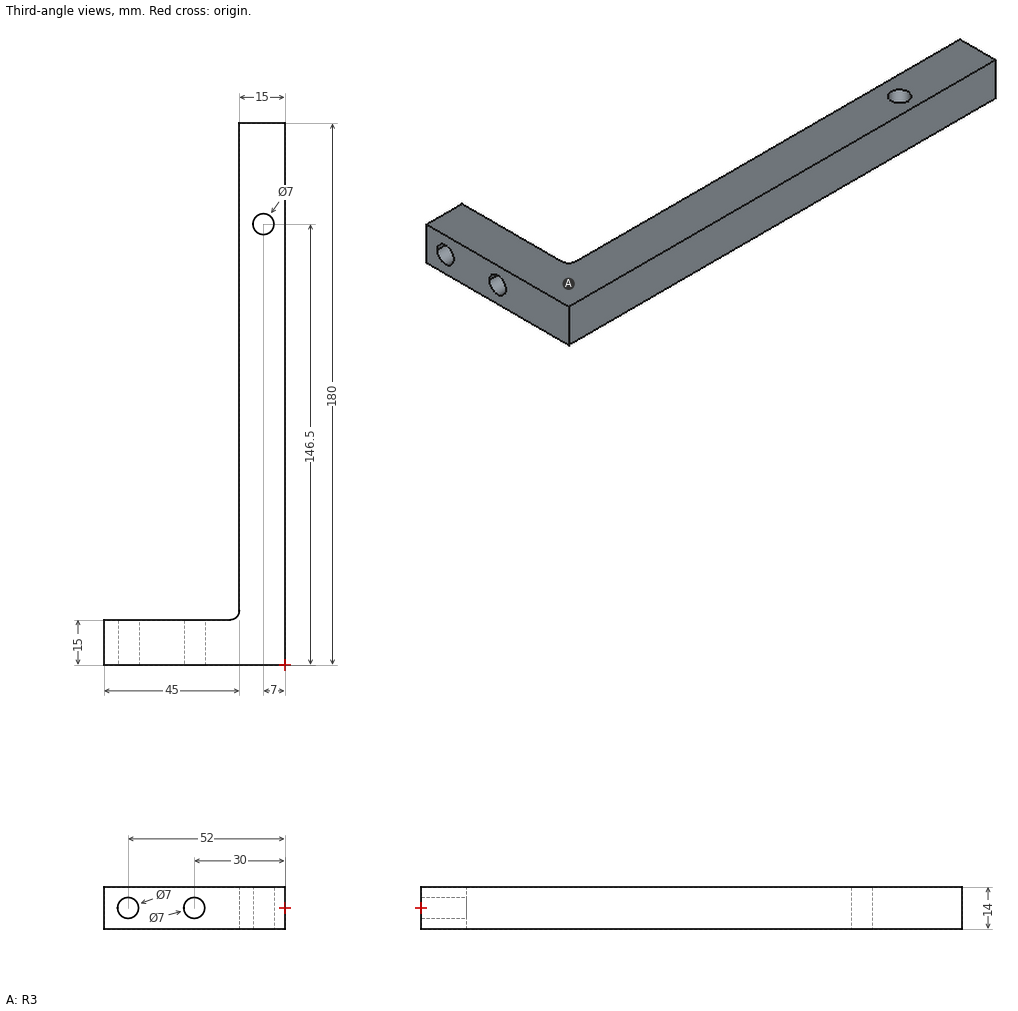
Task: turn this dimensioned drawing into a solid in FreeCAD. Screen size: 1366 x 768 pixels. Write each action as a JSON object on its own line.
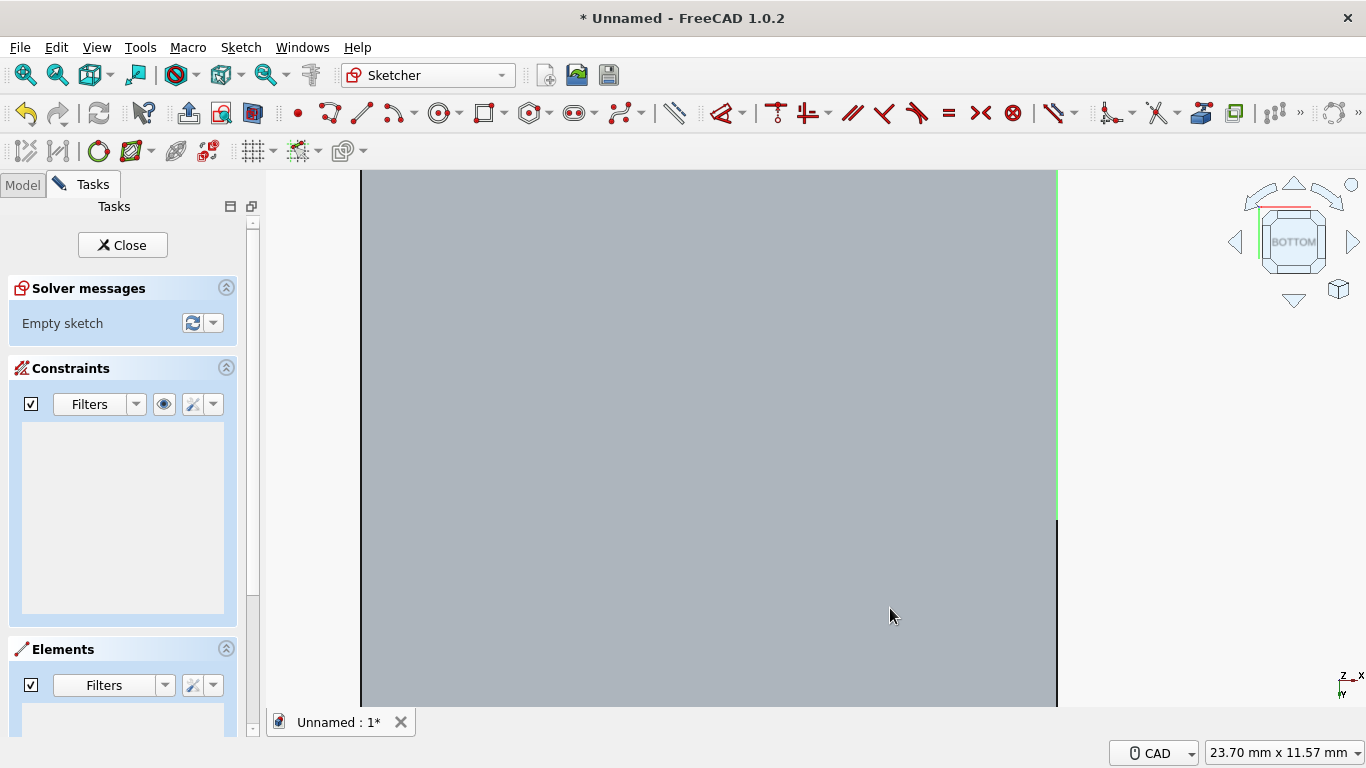
{"action": "left_click", "coordinate": [440, 114]}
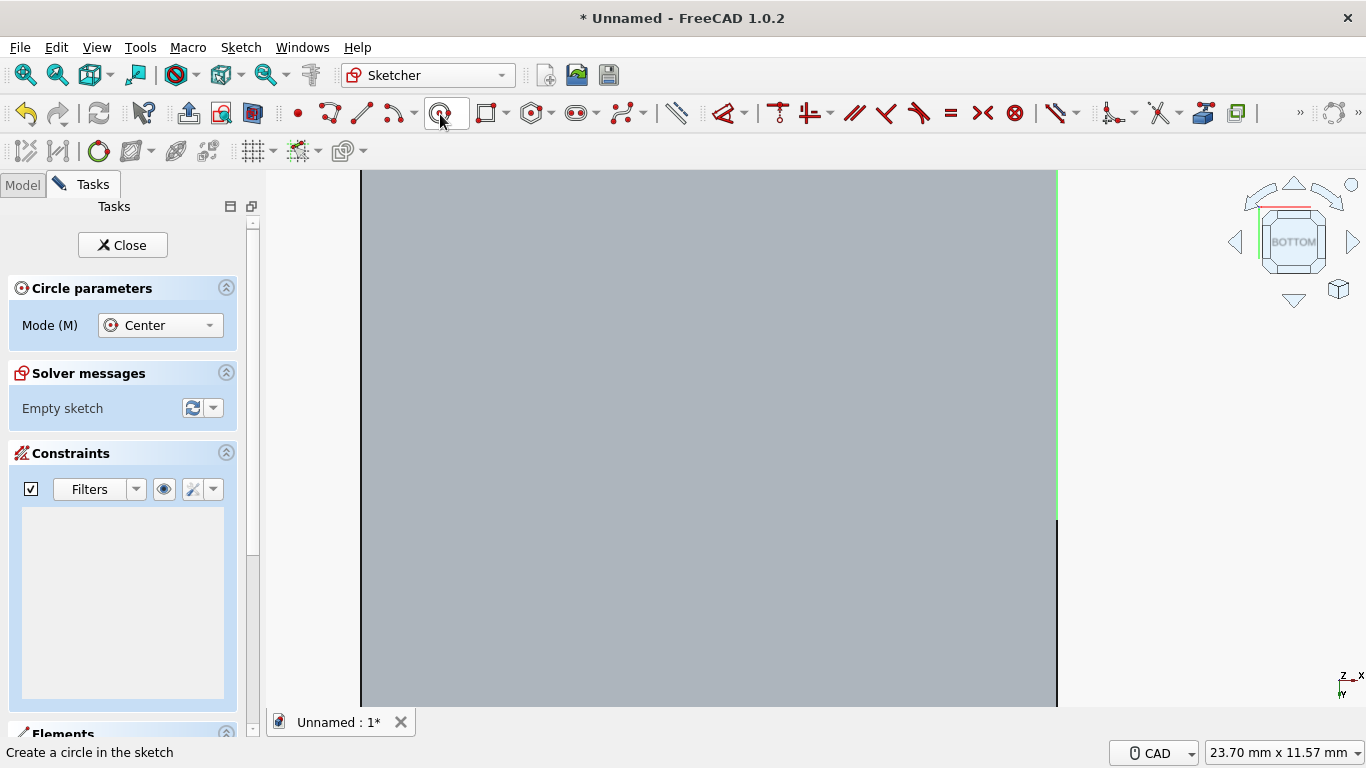
{"action": "left_click", "coordinate": [732, 431]}
{"action": "mouse_move", "coordinate": [847, 316]}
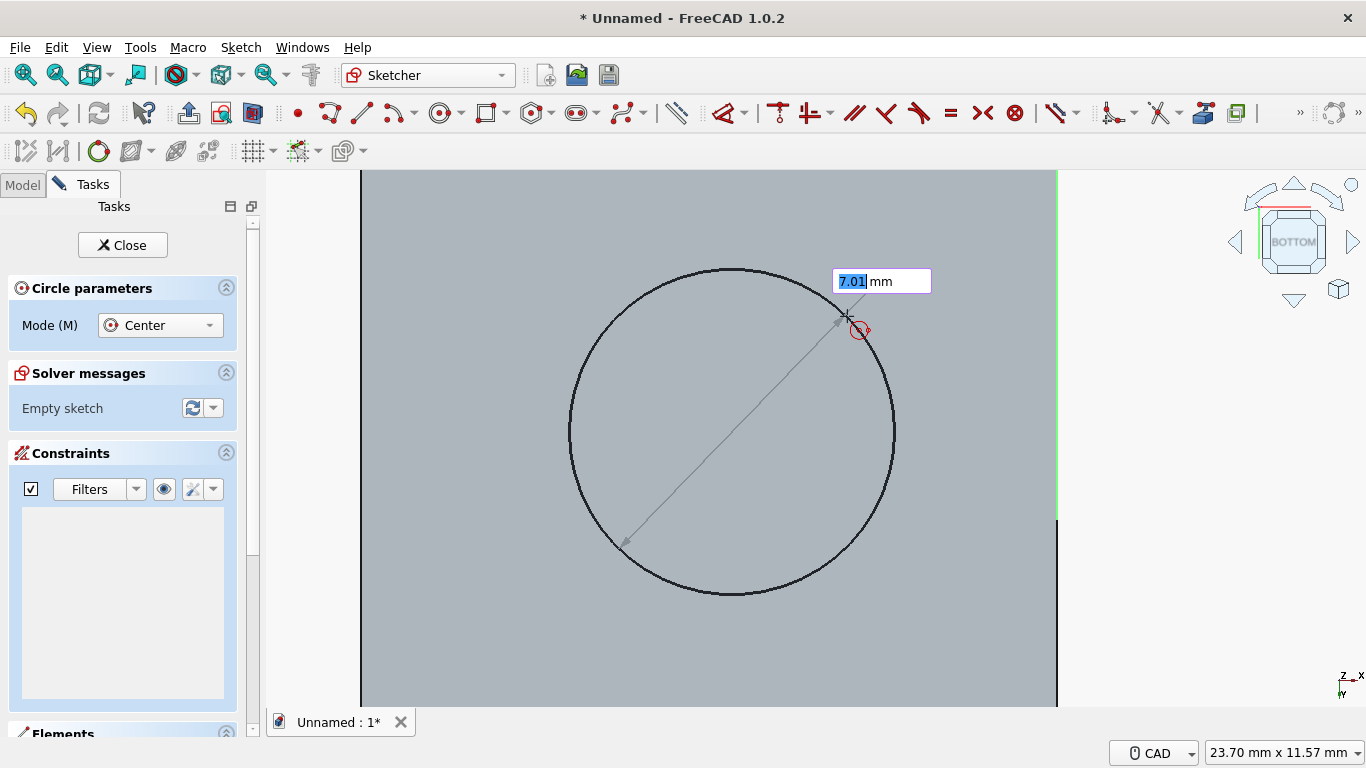
{"action": "type", "text": "7"}
{"action": "key", "text": "Return"}
{"action": "key", "text": "Escape"}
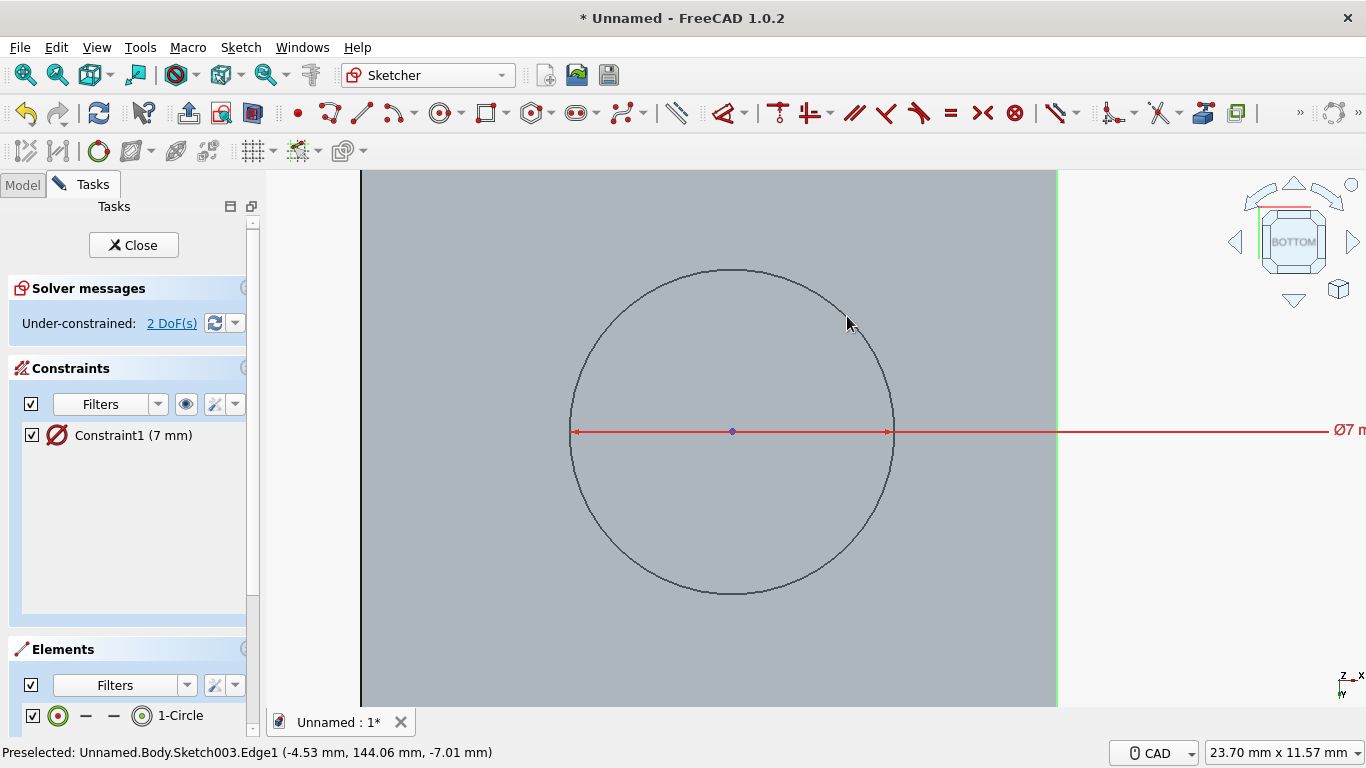
{"action": "left_click", "coordinate": [724, 114]}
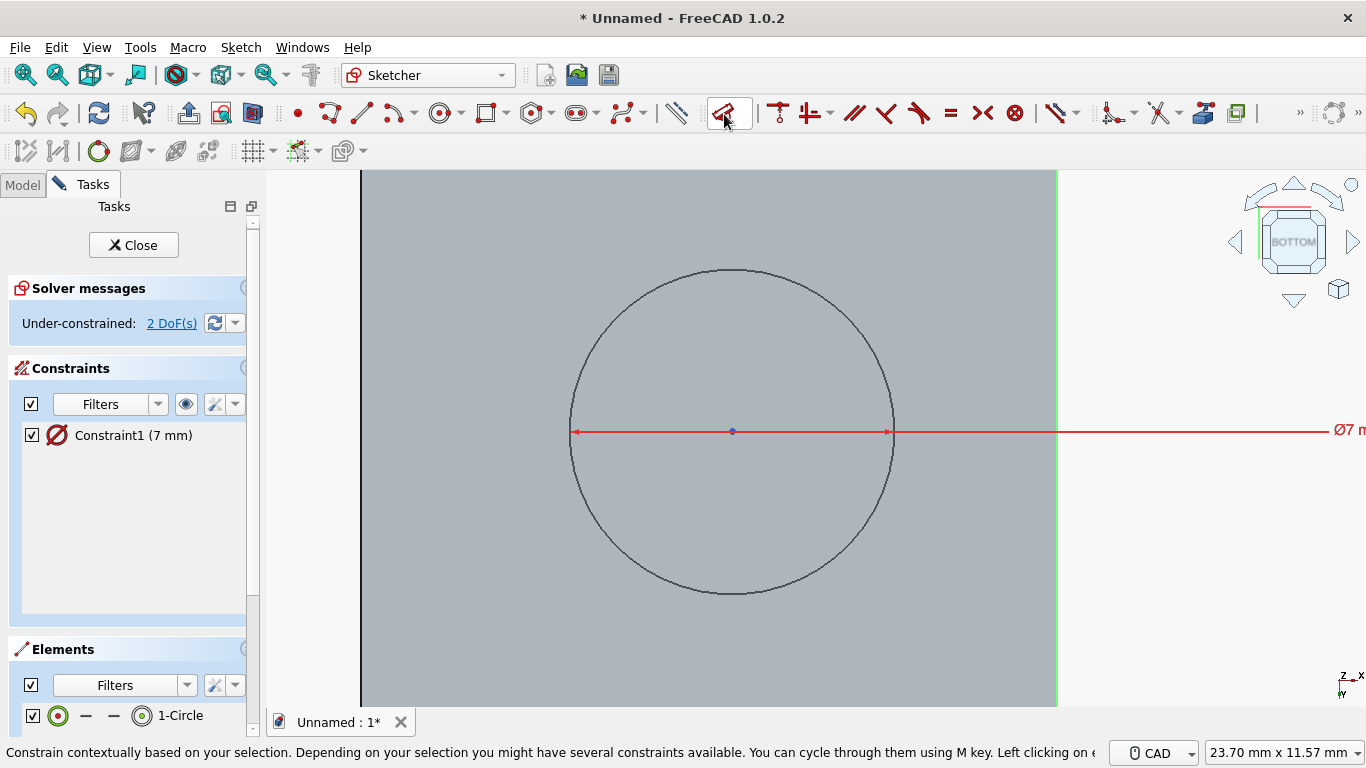
{"action": "left_click", "coordinate": [732, 432]}
{"action": "left_click", "coordinate": [820, 466]}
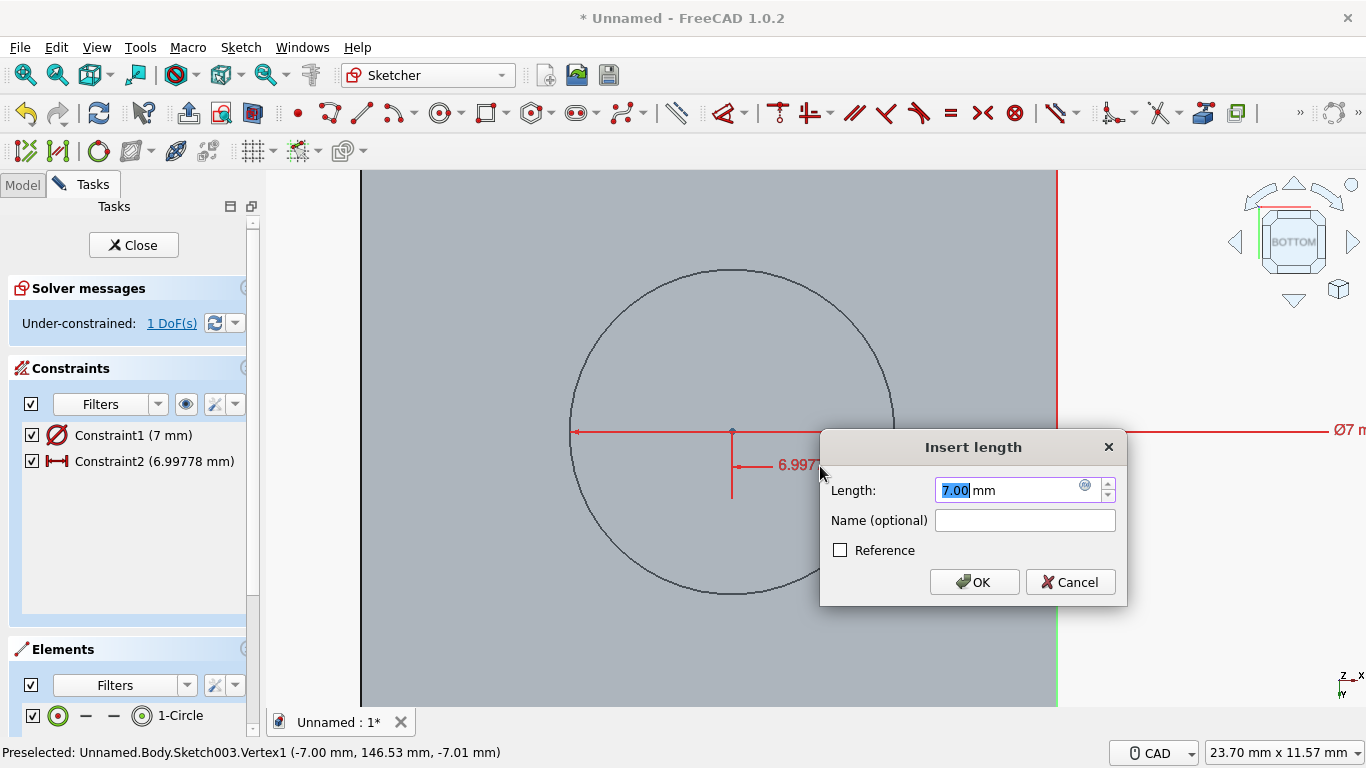
{"action": "type", "text": "7"}
{"action": "key", "text": "Return"}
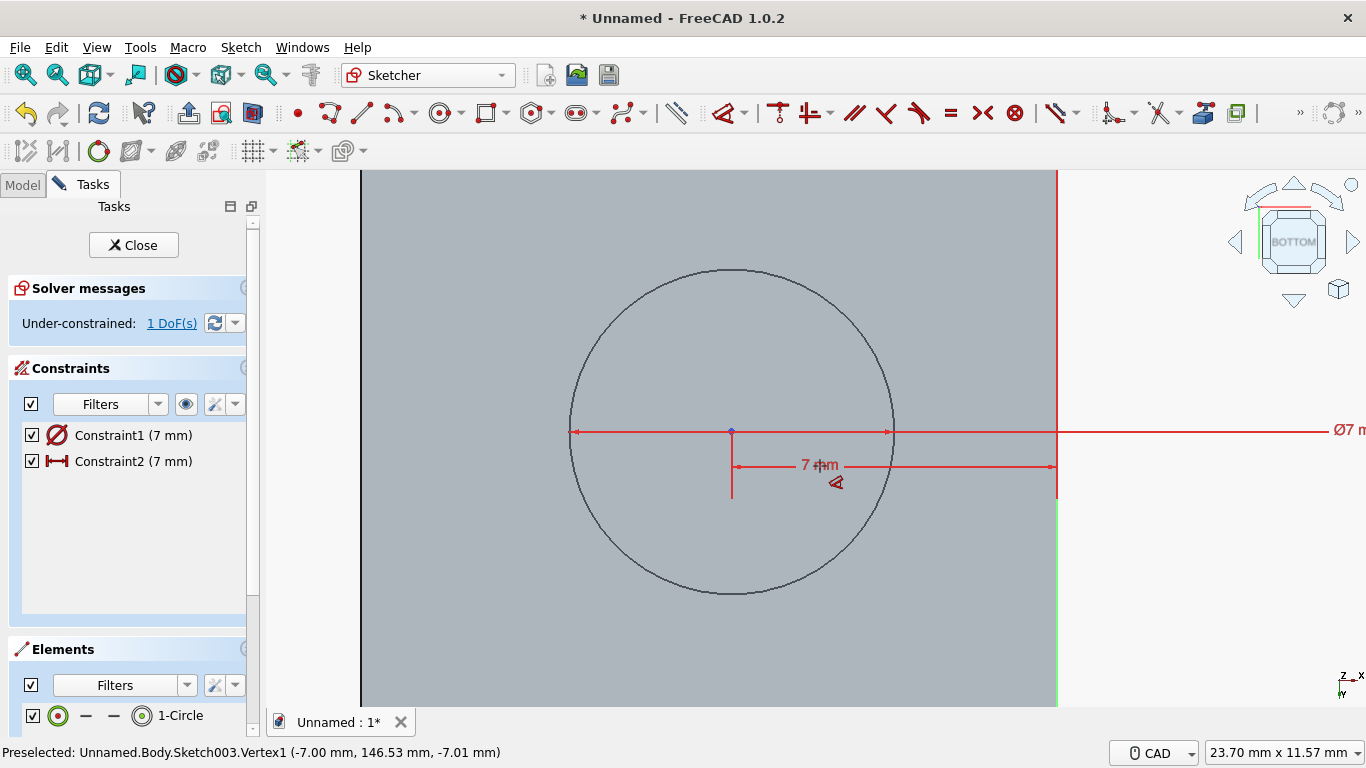
{"action": "left_click", "coordinate": [732, 432]}
{"action": "left_click", "coordinate": [1091, 315]}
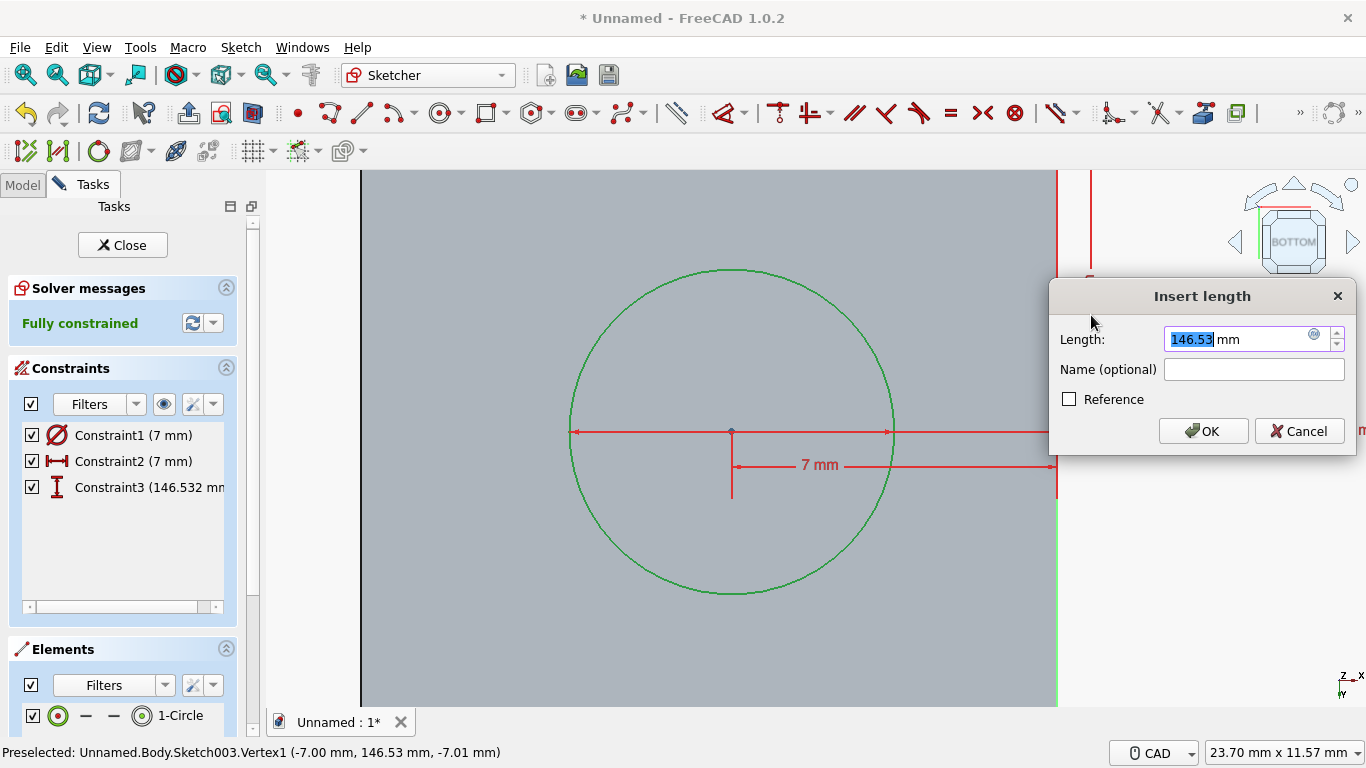
{"action": "type", "text": "146.5"}
{"action": "key", "text": "Return"}
{"action": "key", "text": "Escape"}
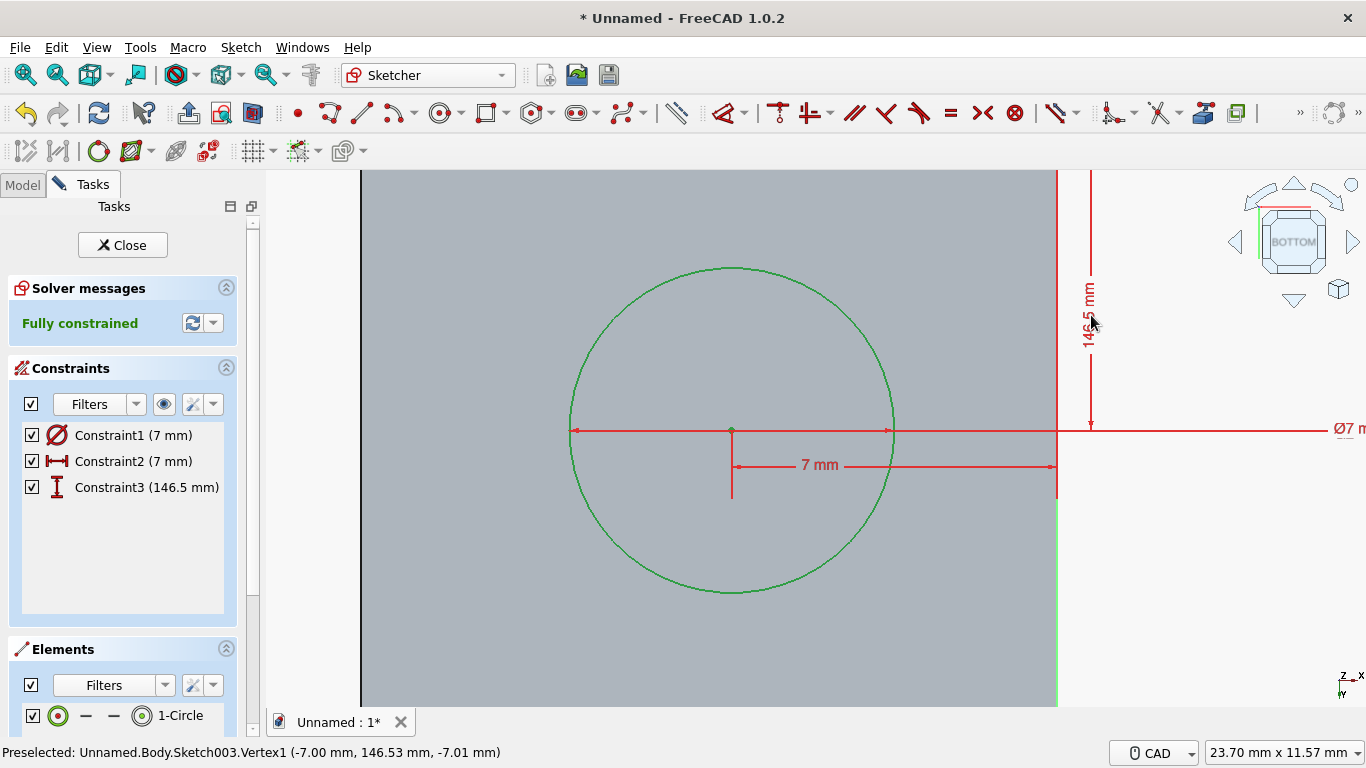
{"action": "left_click", "coordinate": [123, 245]}